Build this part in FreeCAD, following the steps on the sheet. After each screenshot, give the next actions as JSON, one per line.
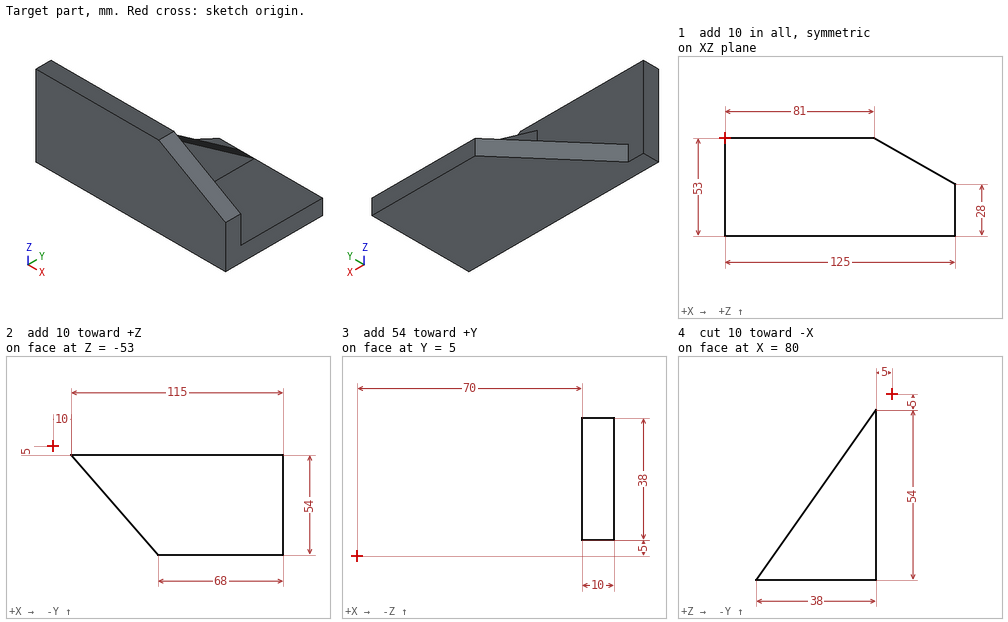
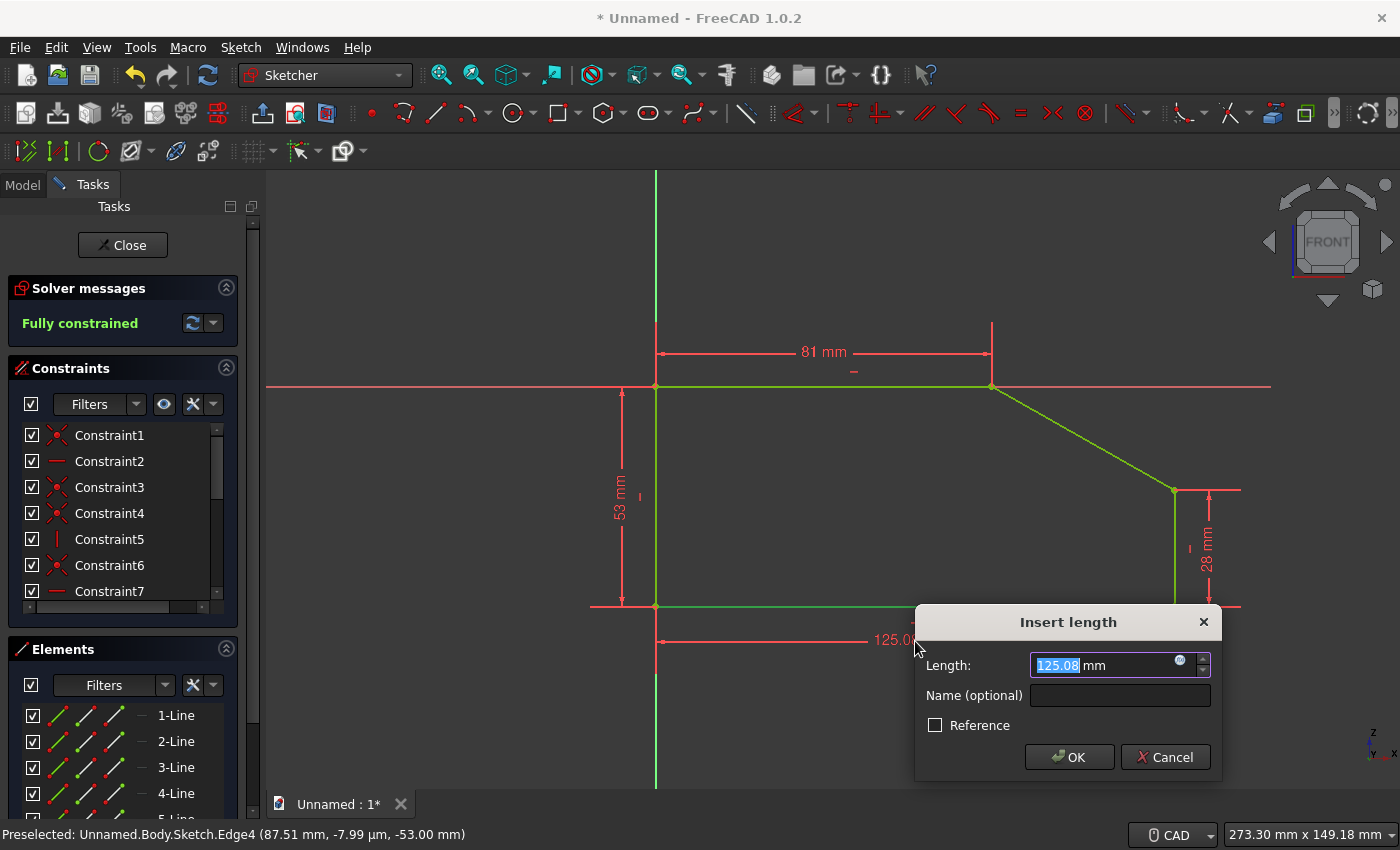
{"action": "type", "text": "125"}
{"action": "key", "text": "Return"}
{"action": "key", "text": "Escape"}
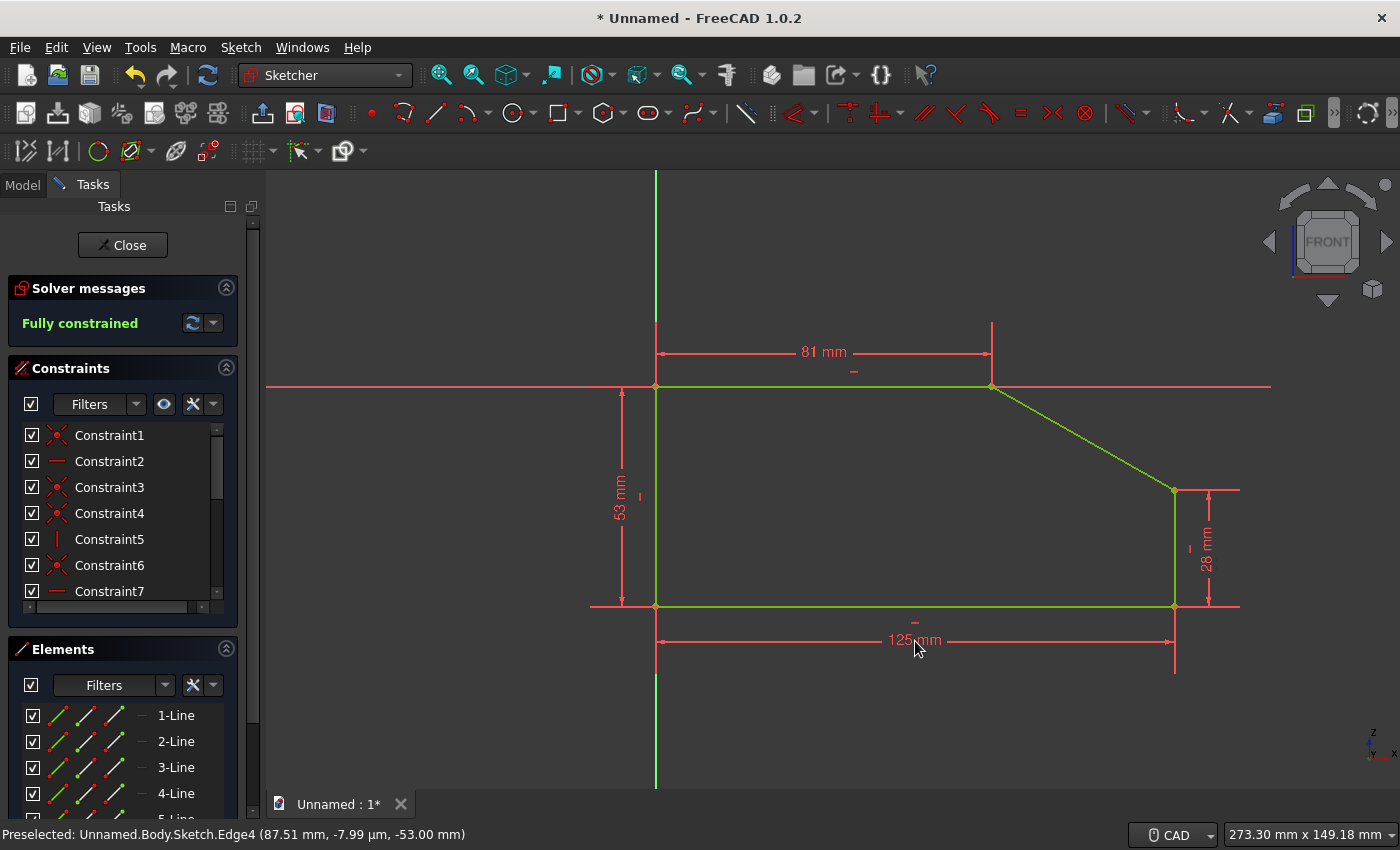
{"action": "left_click", "coordinate": [123, 245]}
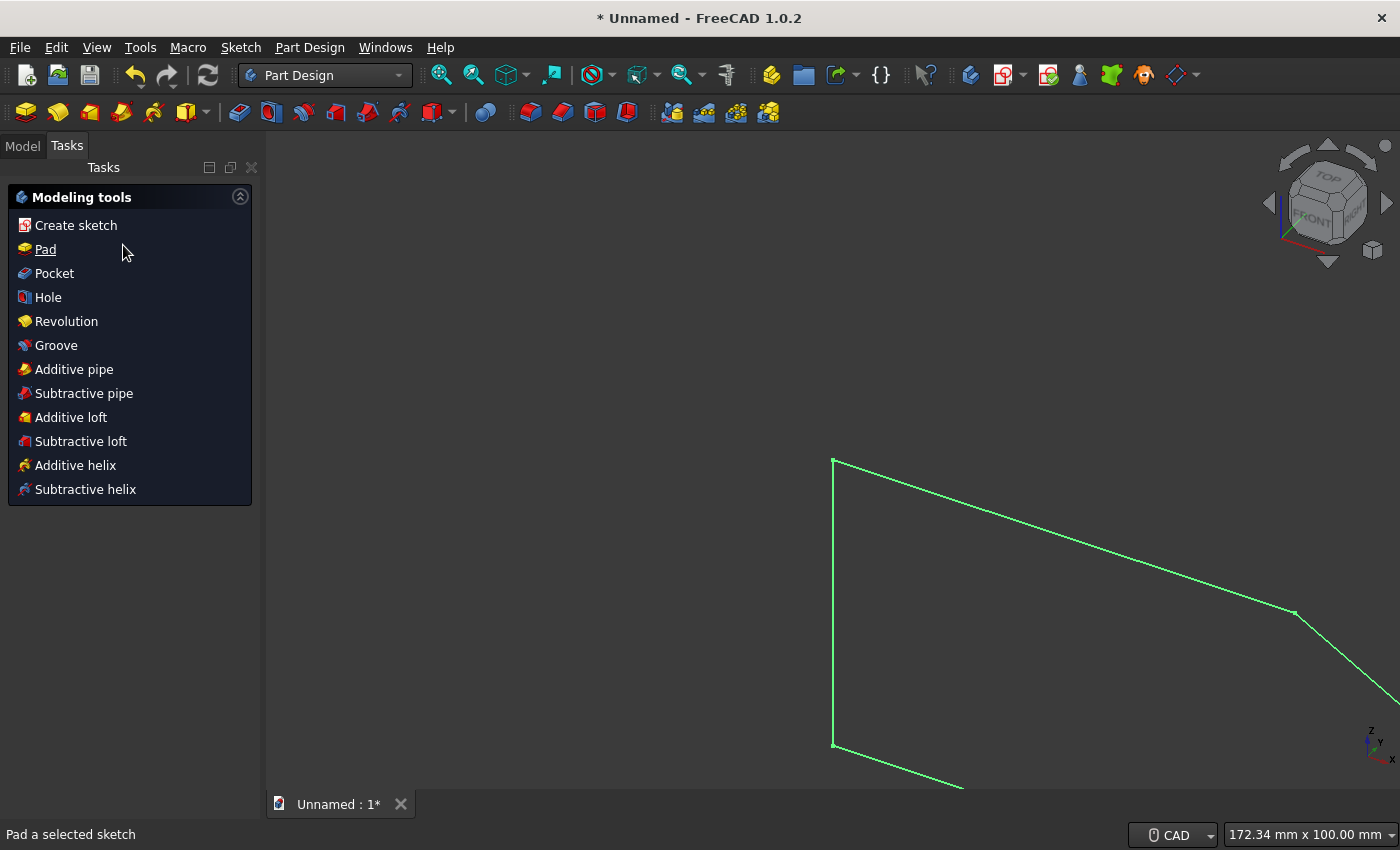
{"action": "left_click", "coordinate": [26, 112]}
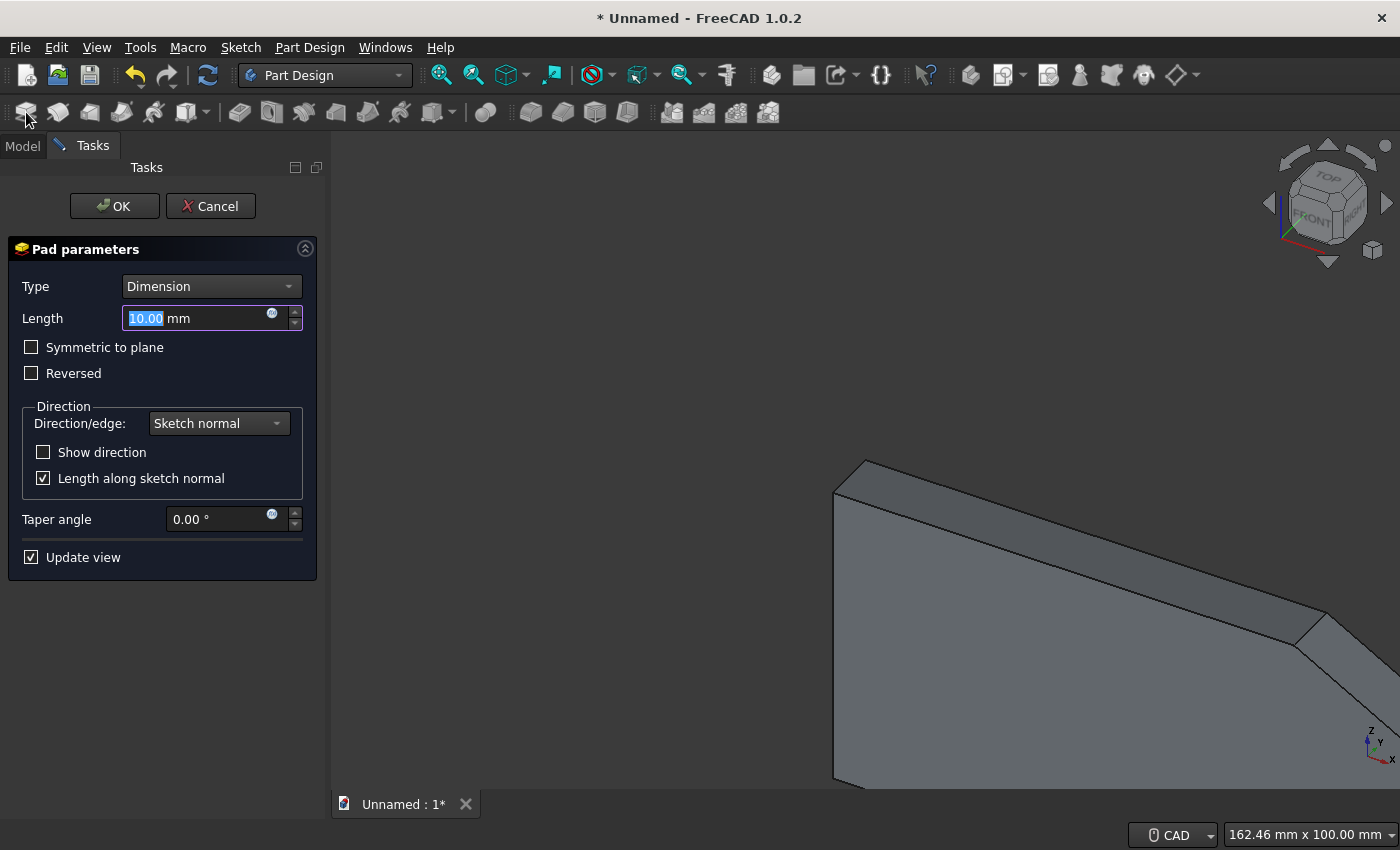
{"action": "type", "text": "10"}
{"action": "key", "text": "Tab"}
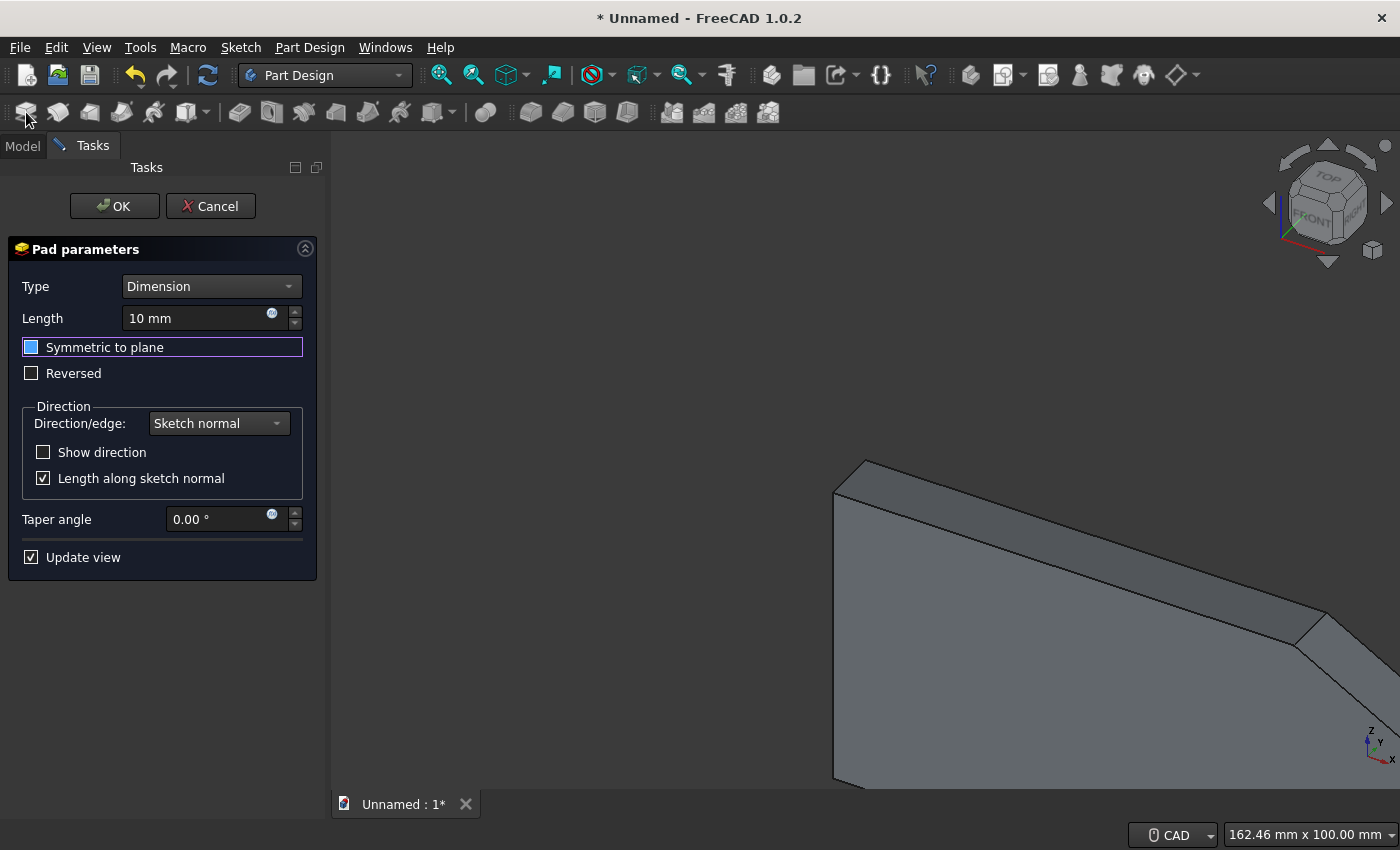
{"action": "left_click", "coordinate": [30, 347]}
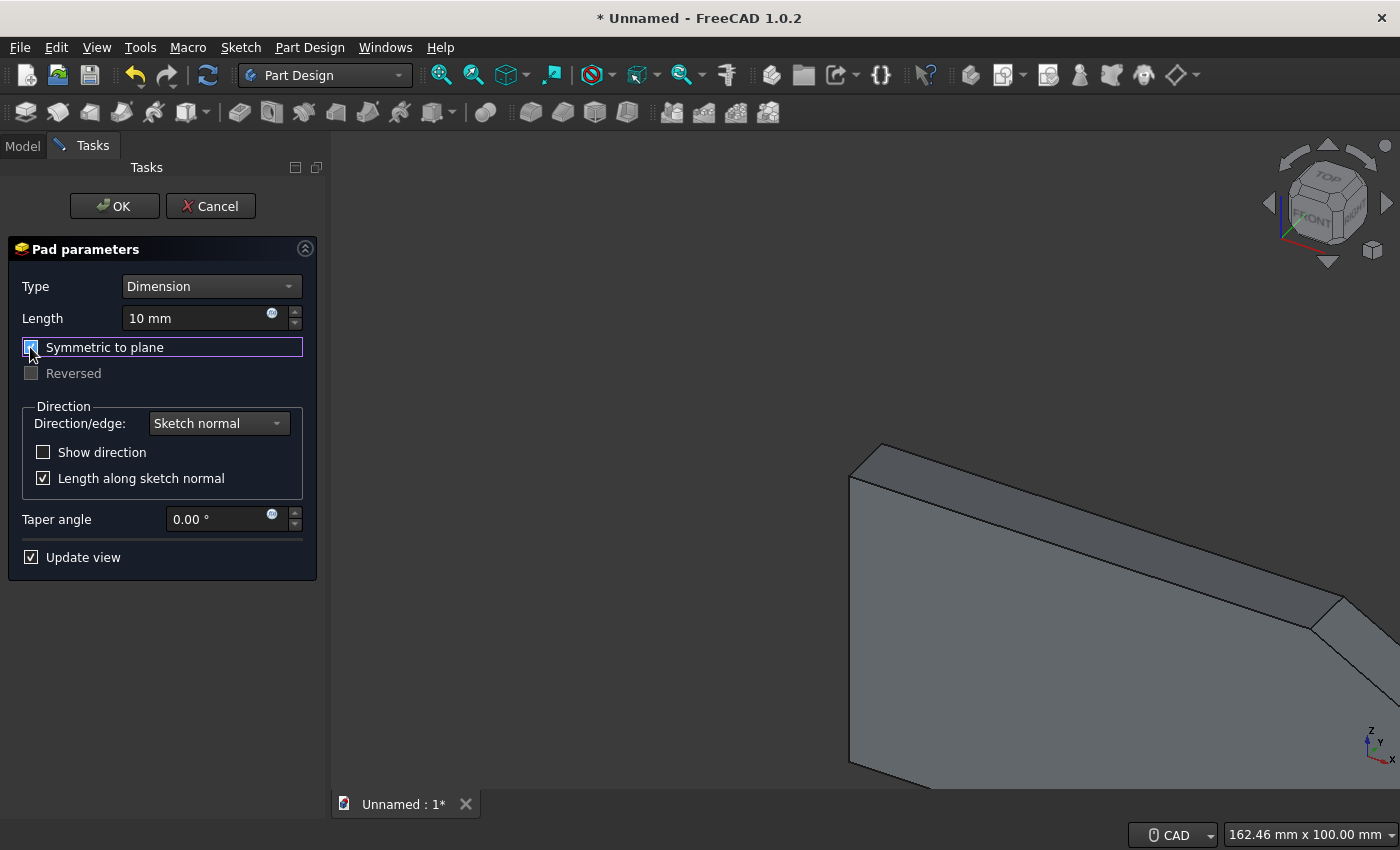
{"action": "left_click", "coordinate": [115, 206]}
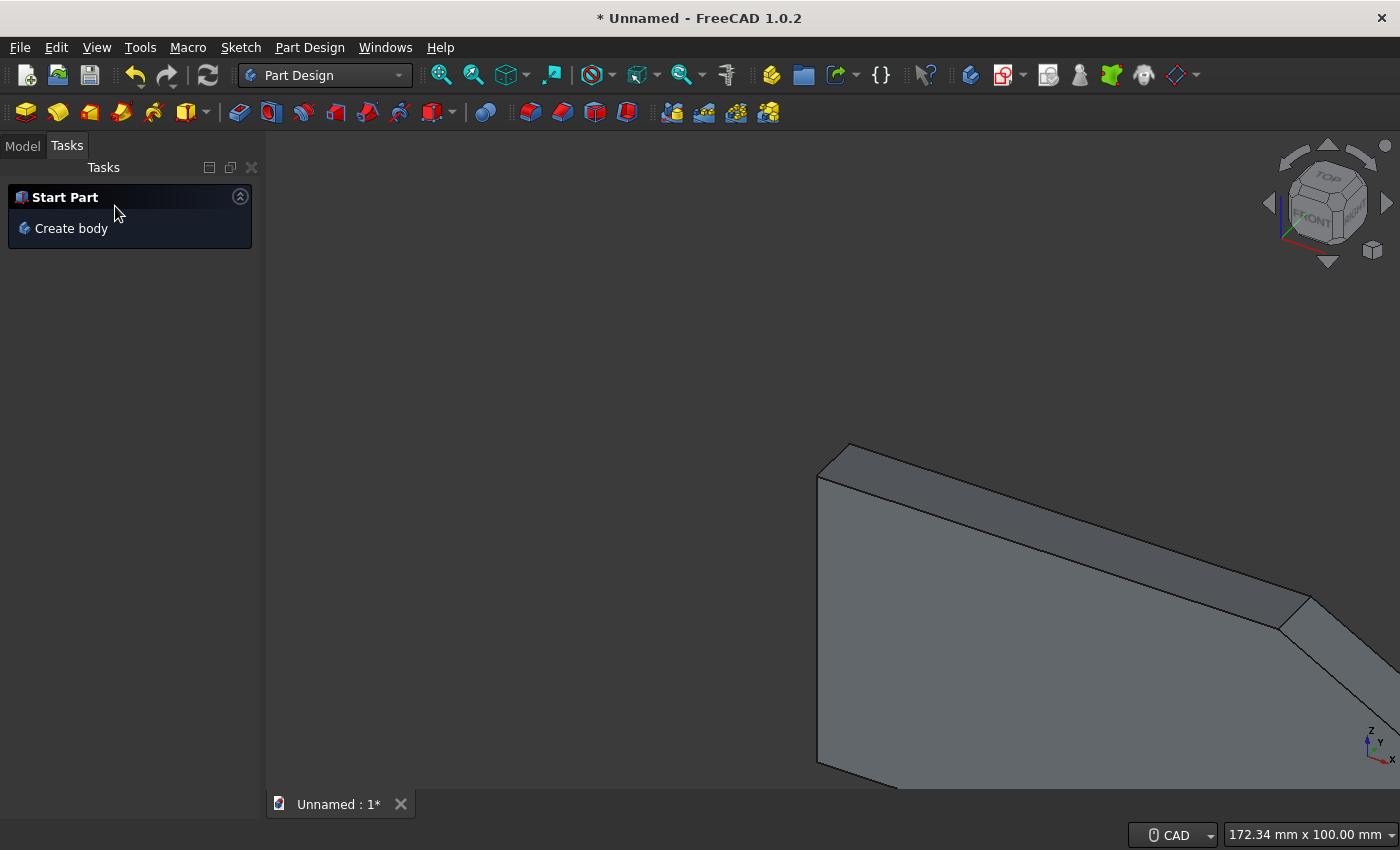
{"action": "key", "text": "v f"}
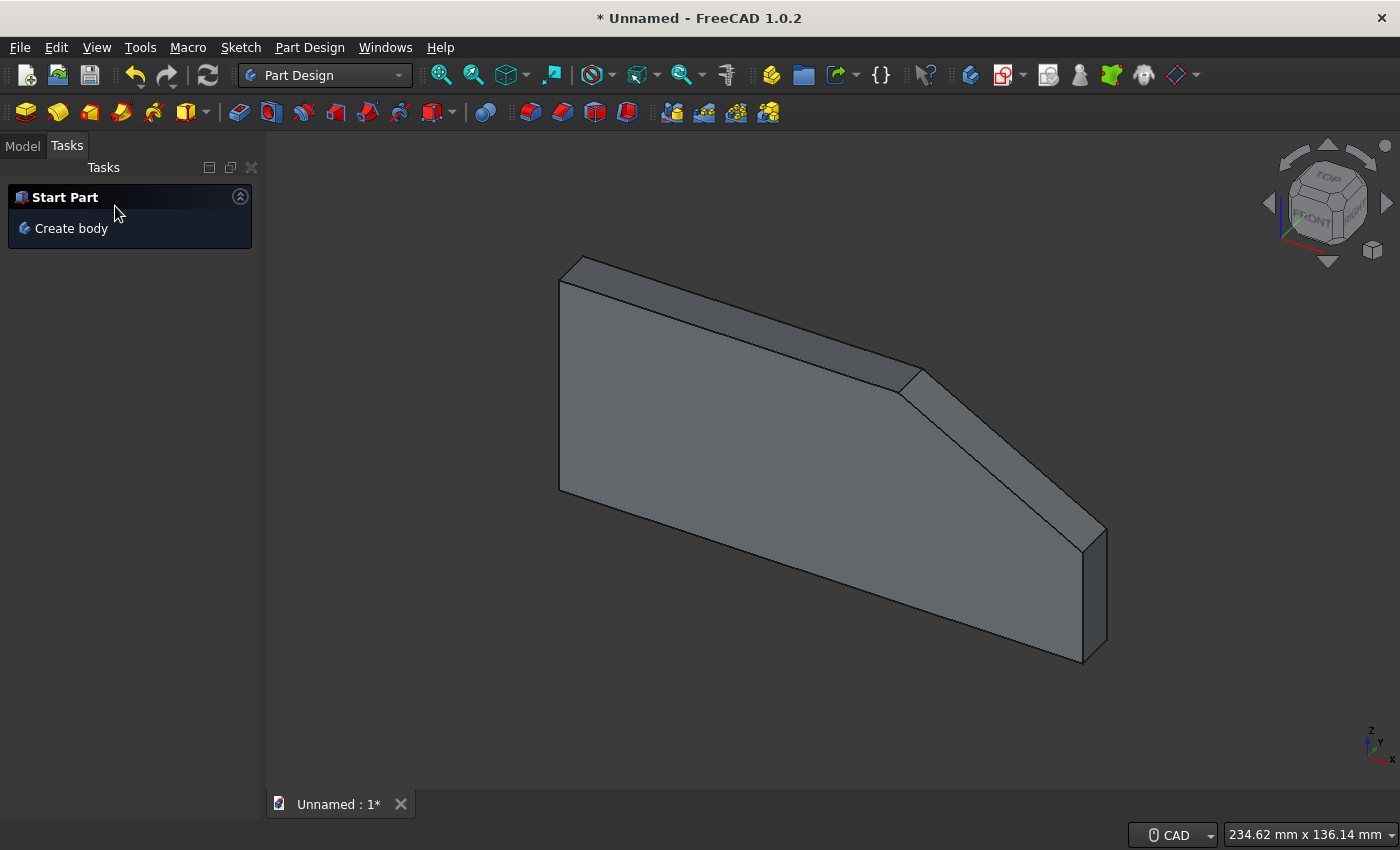
{"action": "key", "text": "5"}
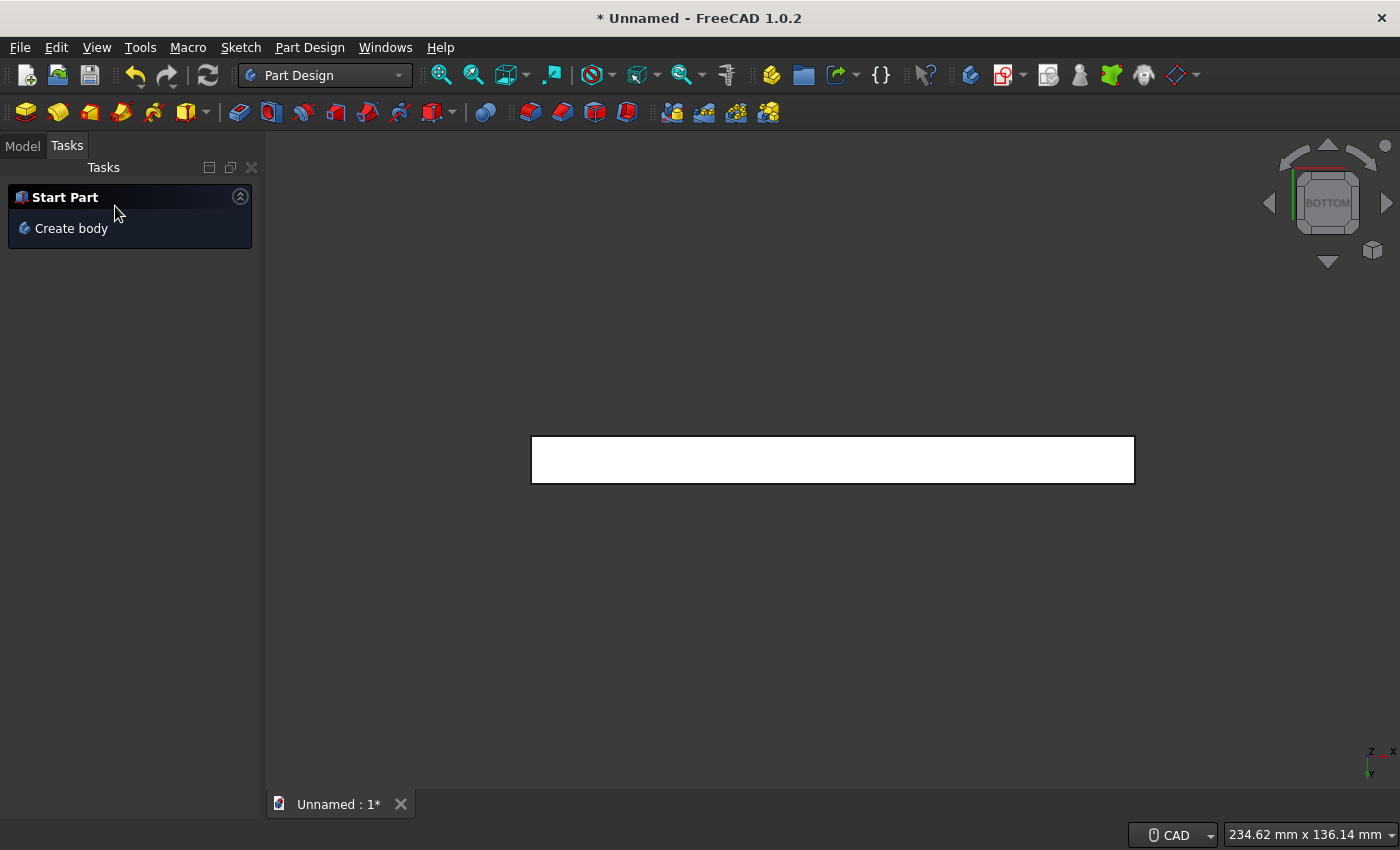
{"action": "left_click", "coordinate": [1092, 459]}